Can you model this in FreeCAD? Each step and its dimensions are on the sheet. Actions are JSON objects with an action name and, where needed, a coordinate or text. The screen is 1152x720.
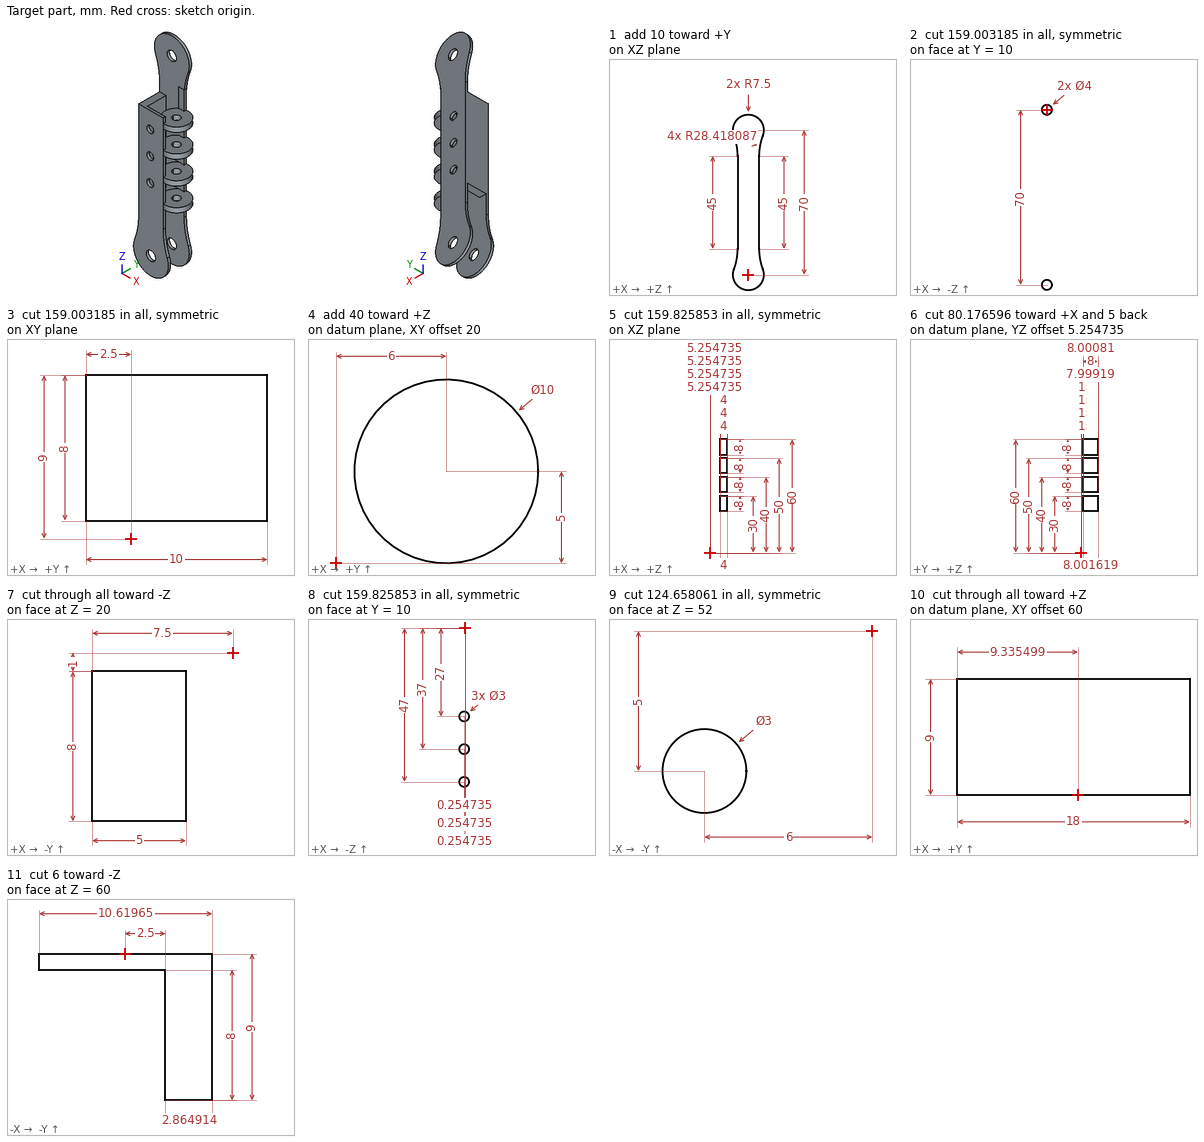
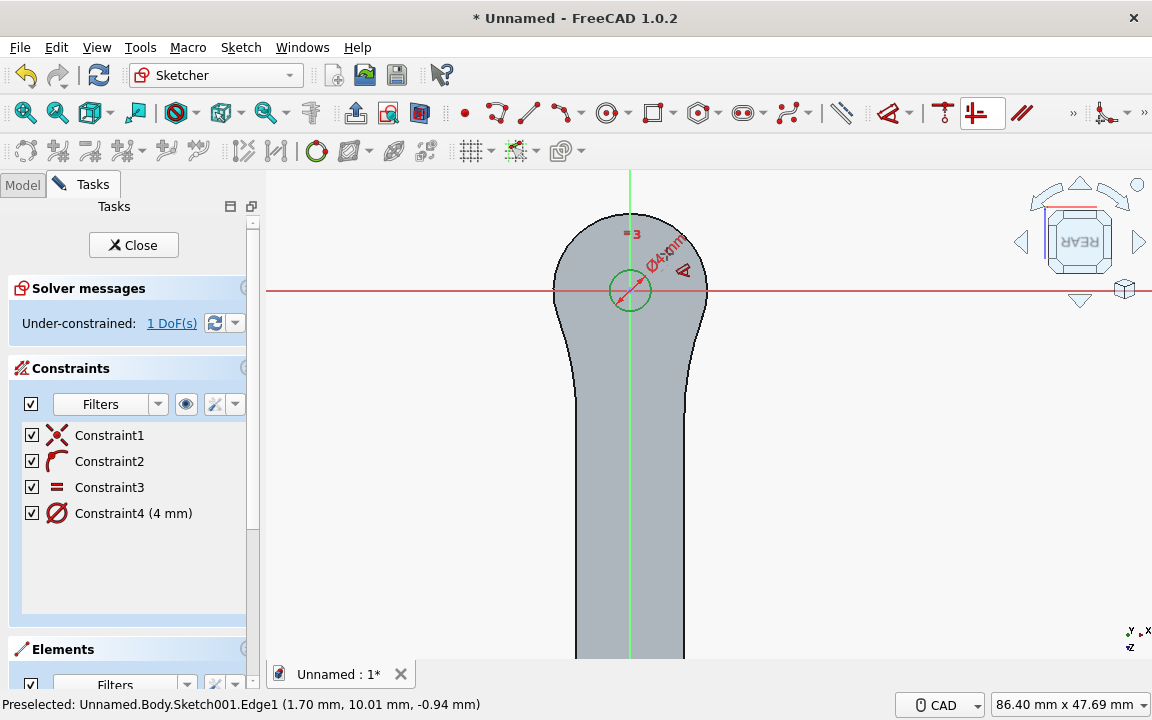
{"action": "scroll", "coordinate": [646, 278], "scroll_direction": "down", "scroll_amount": 5}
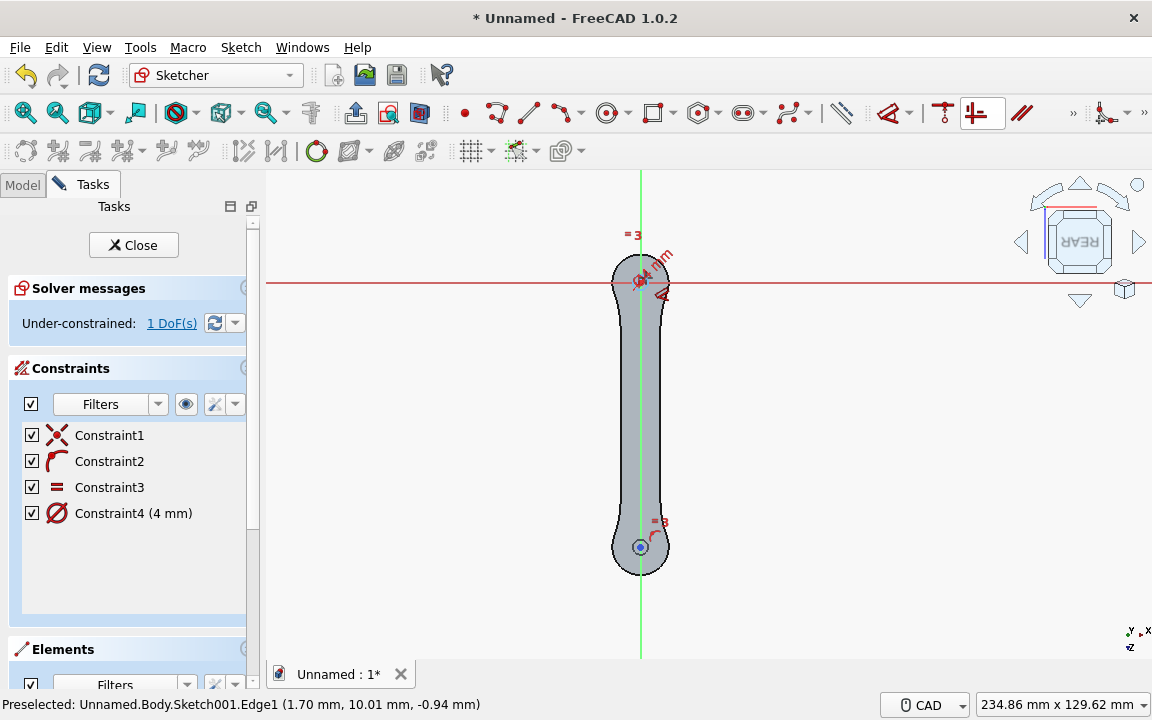
{"action": "left_click", "coordinate": [641, 547]}
{"action": "left_click", "coordinate": [675, 415]}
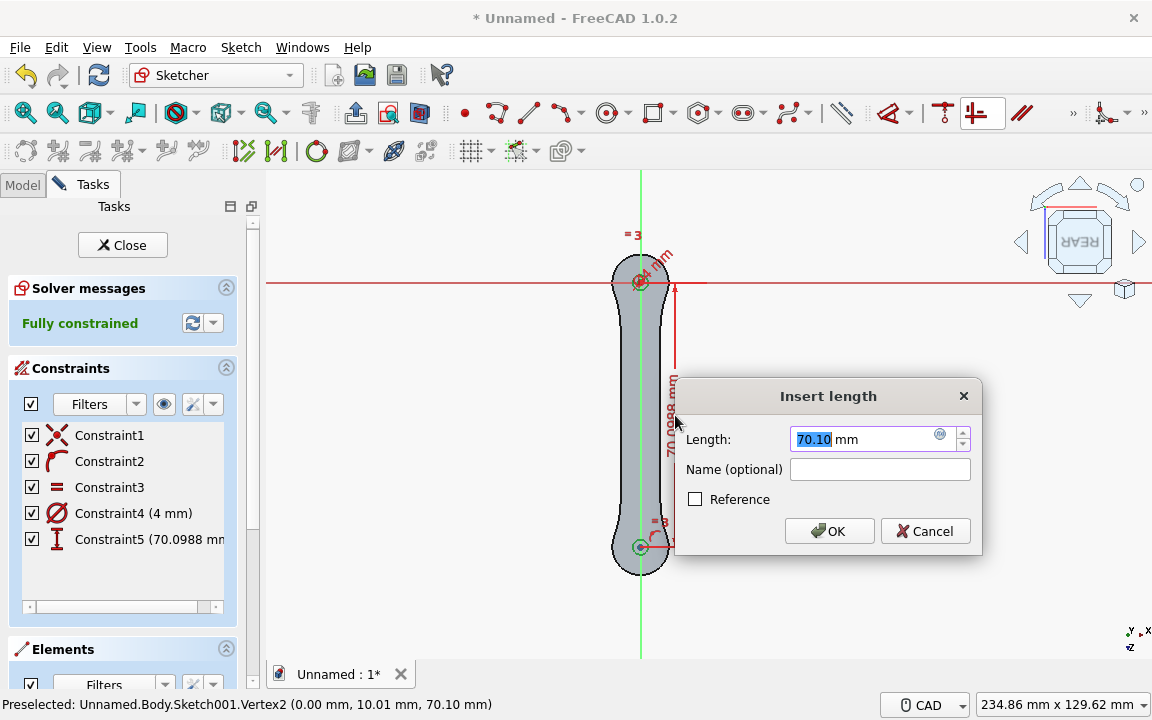
{"action": "type", "text": "70"}
{"action": "key", "text": "Return"}
{"action": "key", "text": "Escape"}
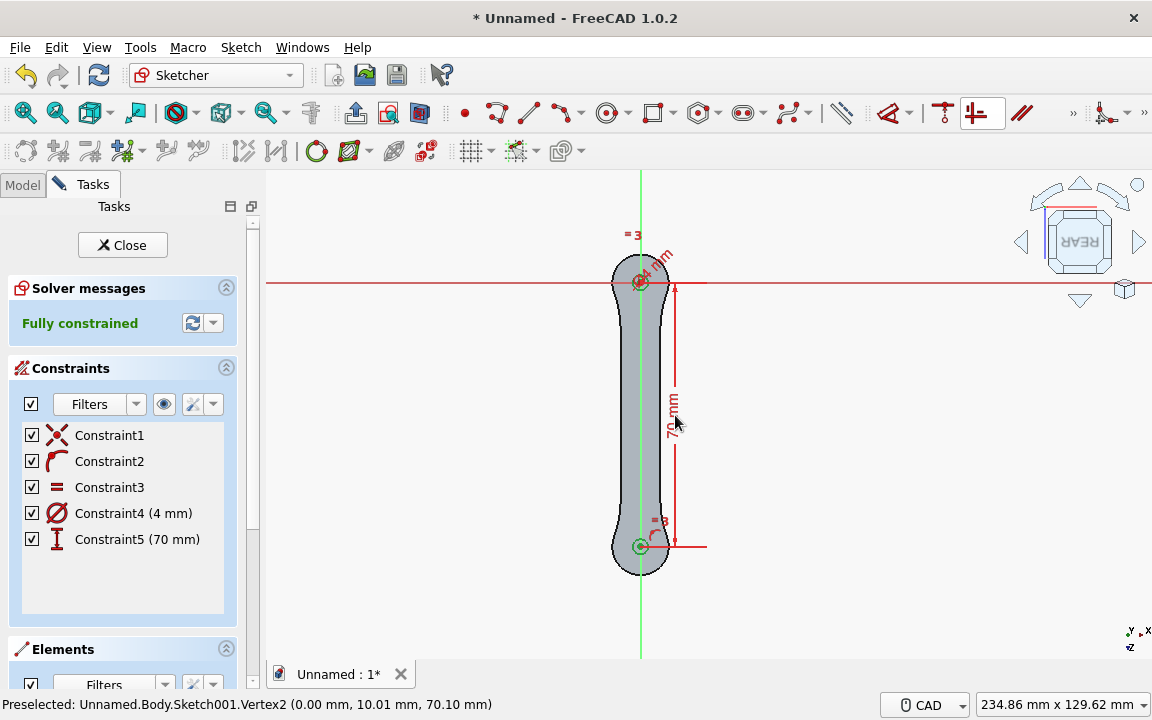
{"action": "left_click", "coordinate": [123, 245]}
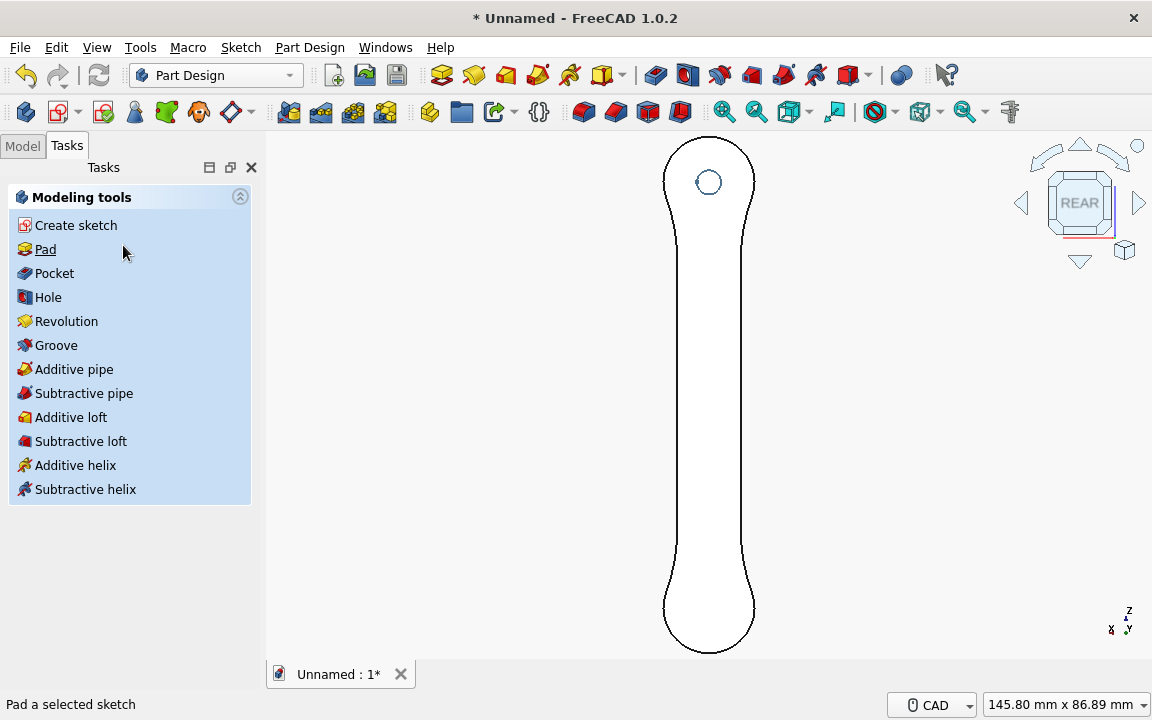
{"action": "left_click", "coordinate": [656, 76]}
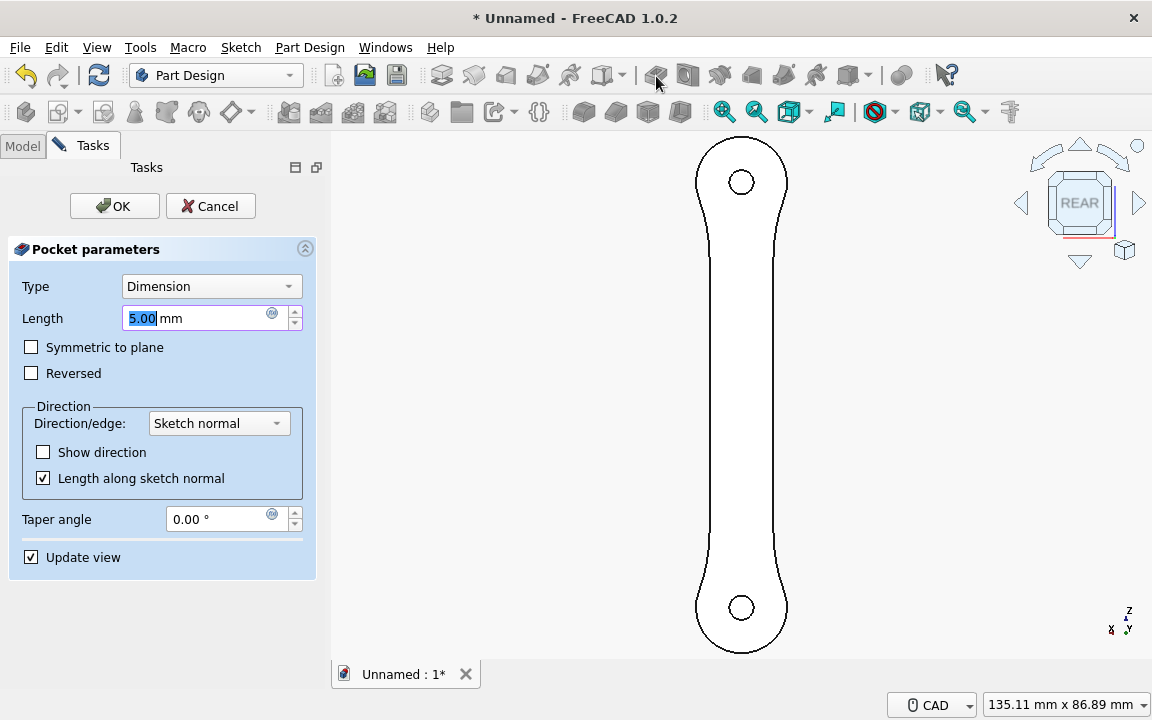
{"action": "type", "text": "159.003185"}
{"action": "key", "text": "Tab"}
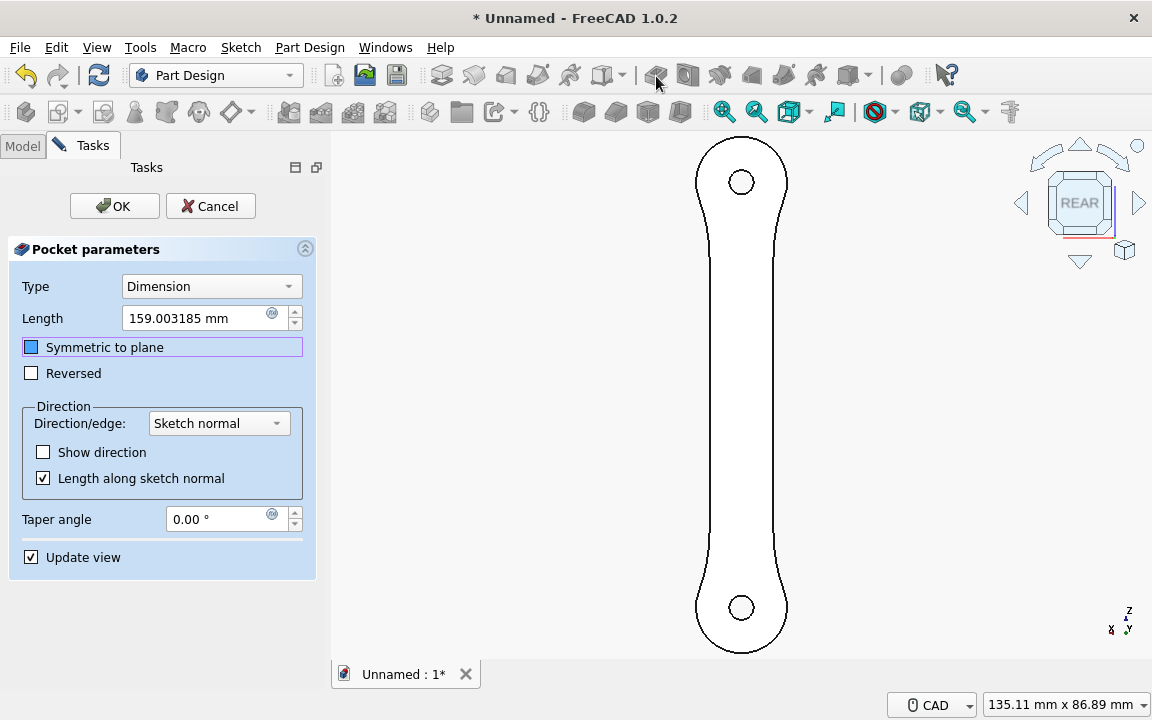
{"action": "left_click", "coordinate": [30, 347]}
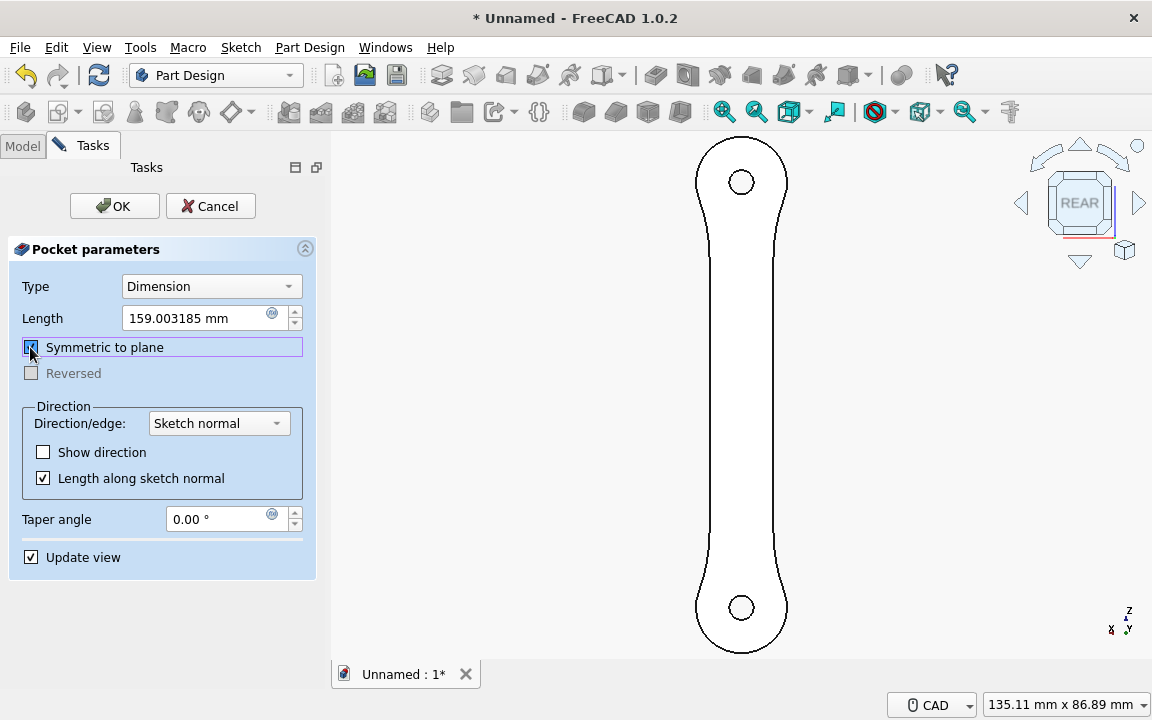
{"action": "left_click", "coordinate": [115, 206]}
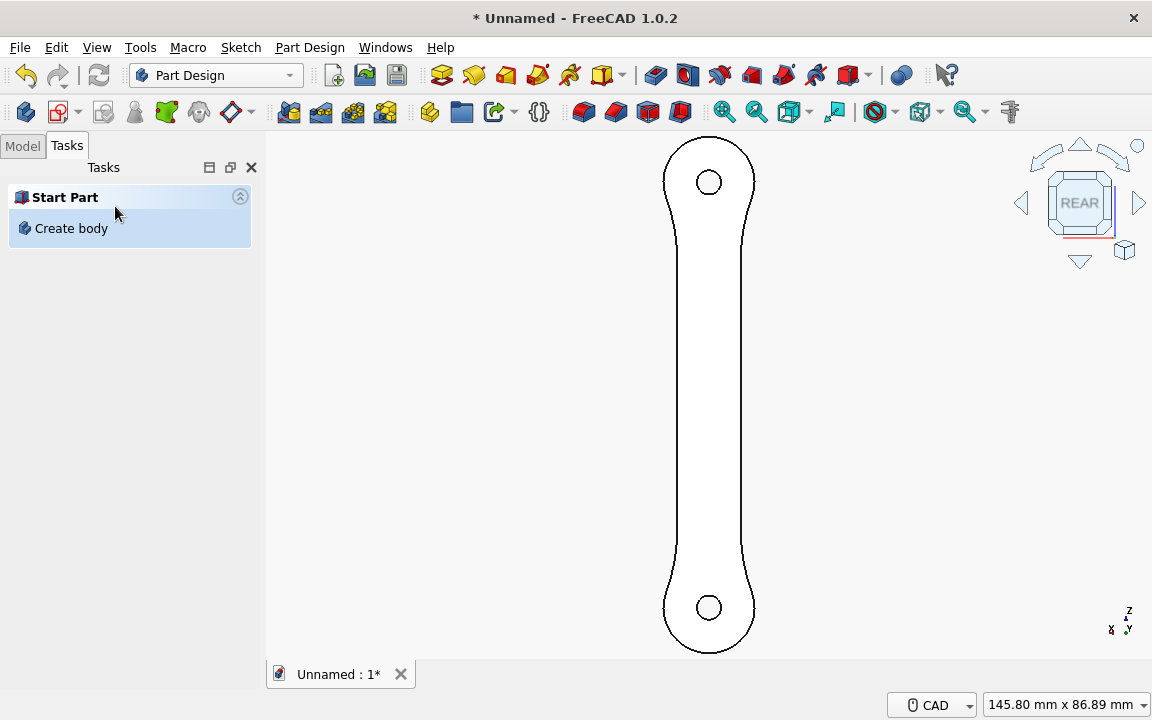
{"action": "left_click", "coordinate": [58, 112]}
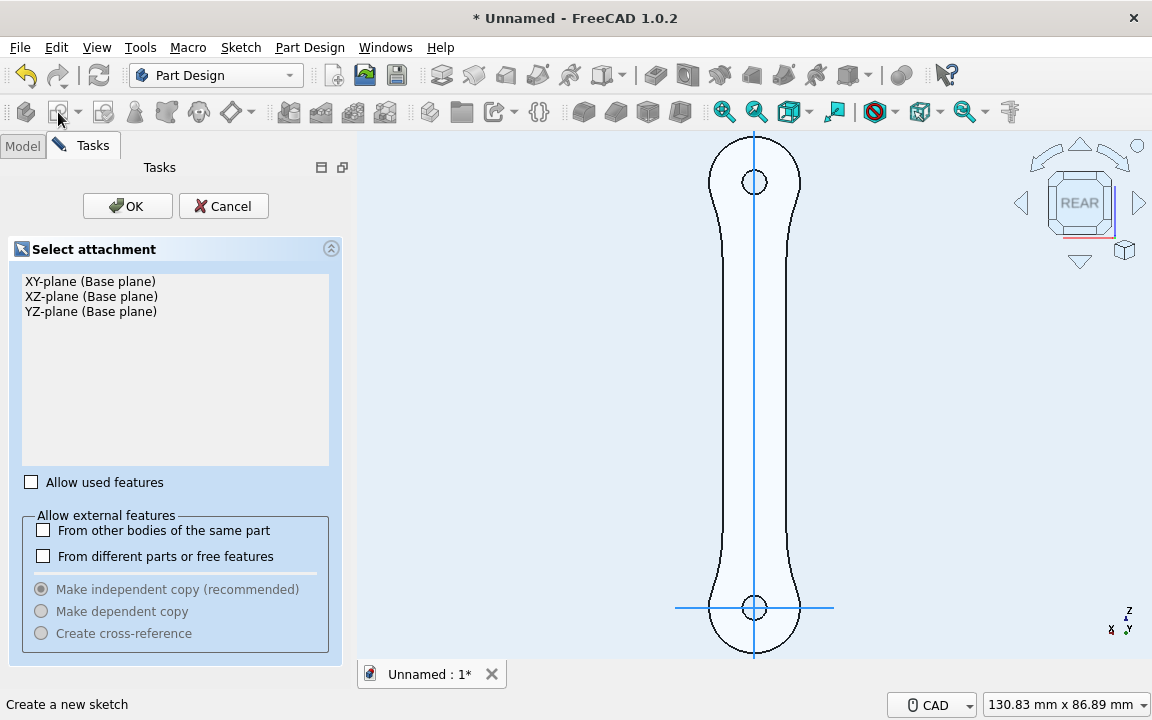
{"action": "left_click", "coordinate": [82, 282]}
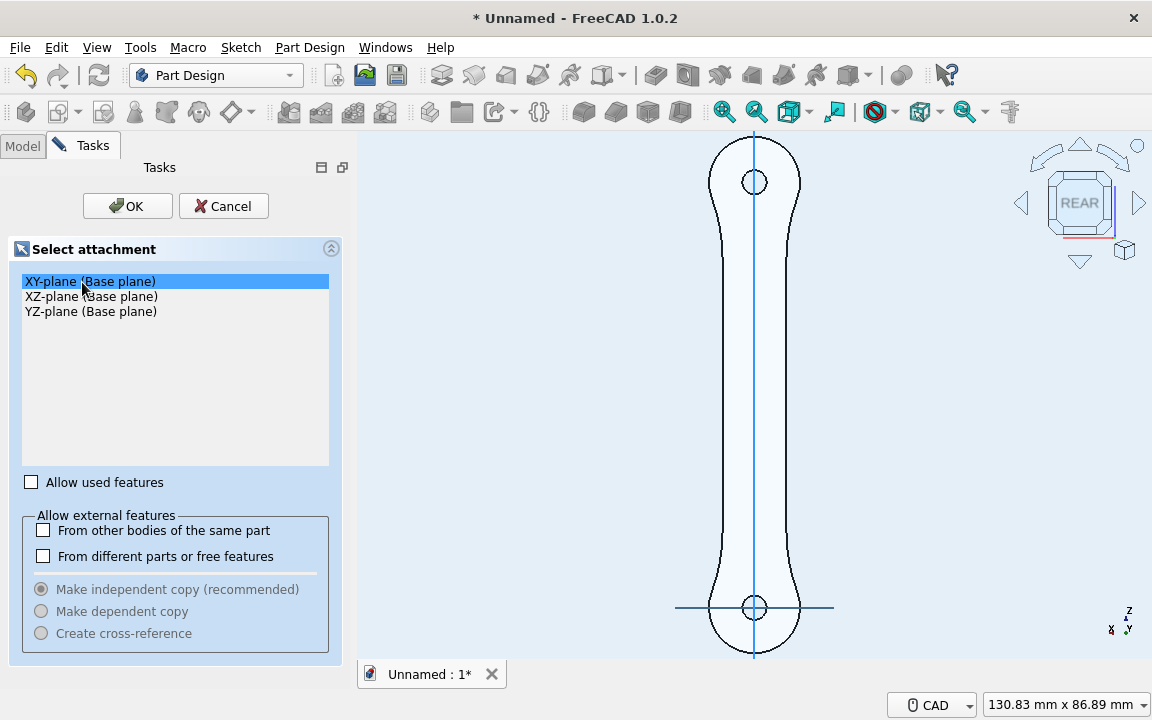
{"action": "left_click", "coordinate": [128, 206]}